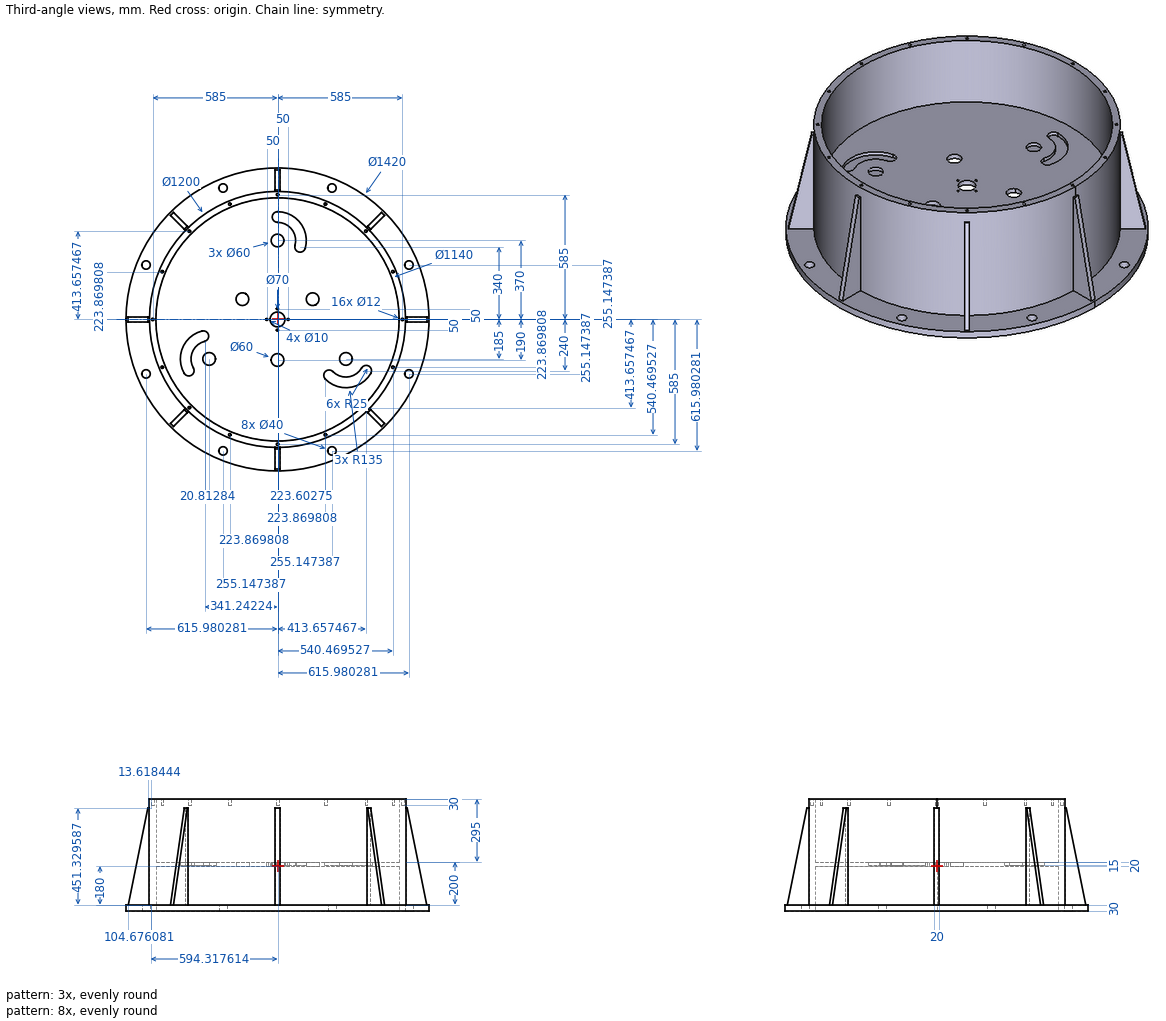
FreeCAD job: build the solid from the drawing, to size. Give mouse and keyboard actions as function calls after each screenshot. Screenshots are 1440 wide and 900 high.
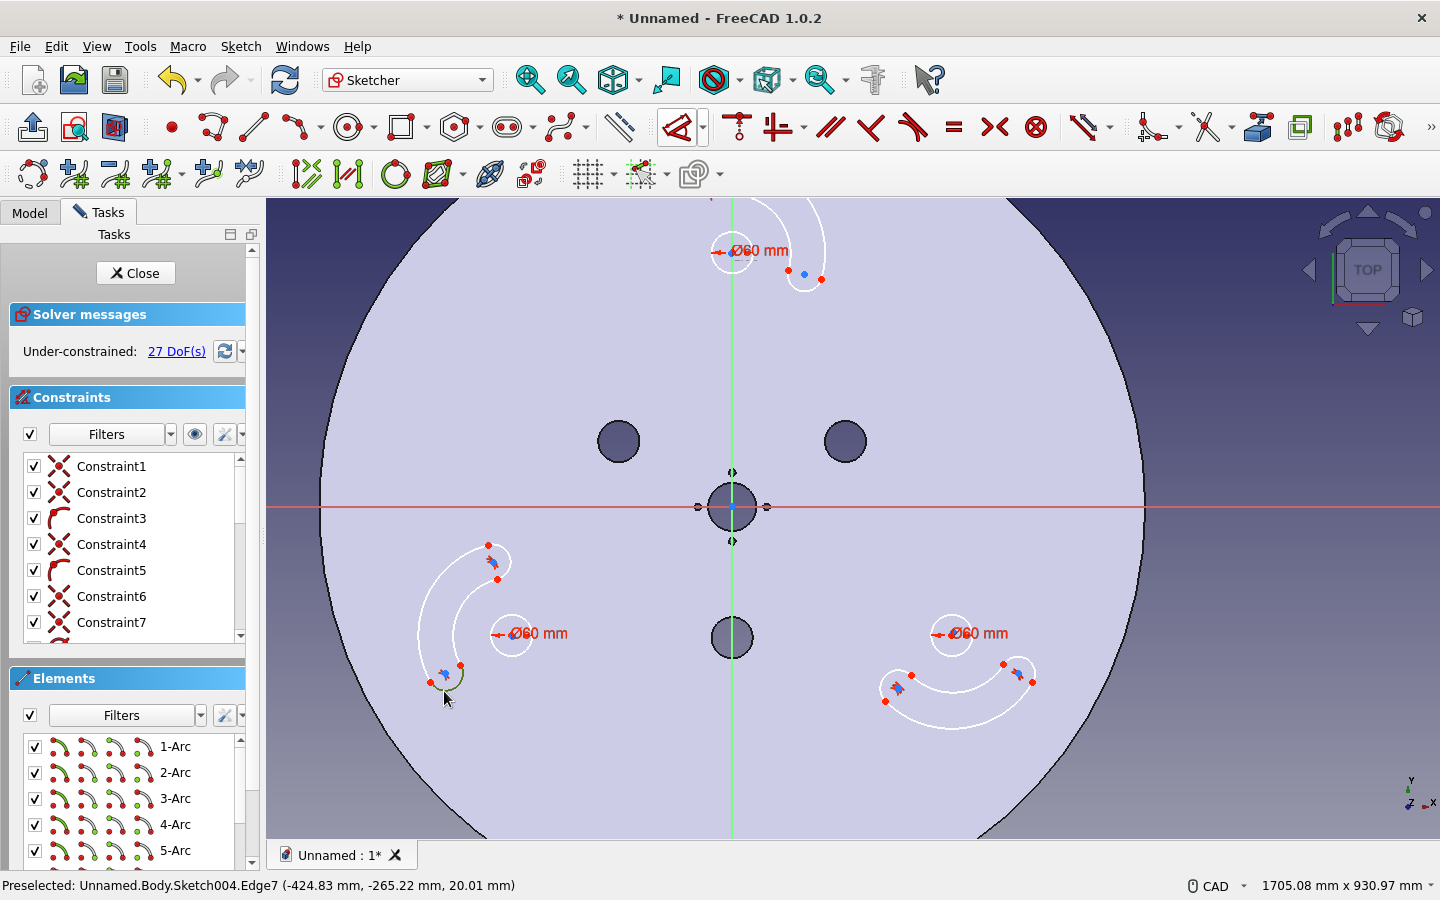
click(470, 595)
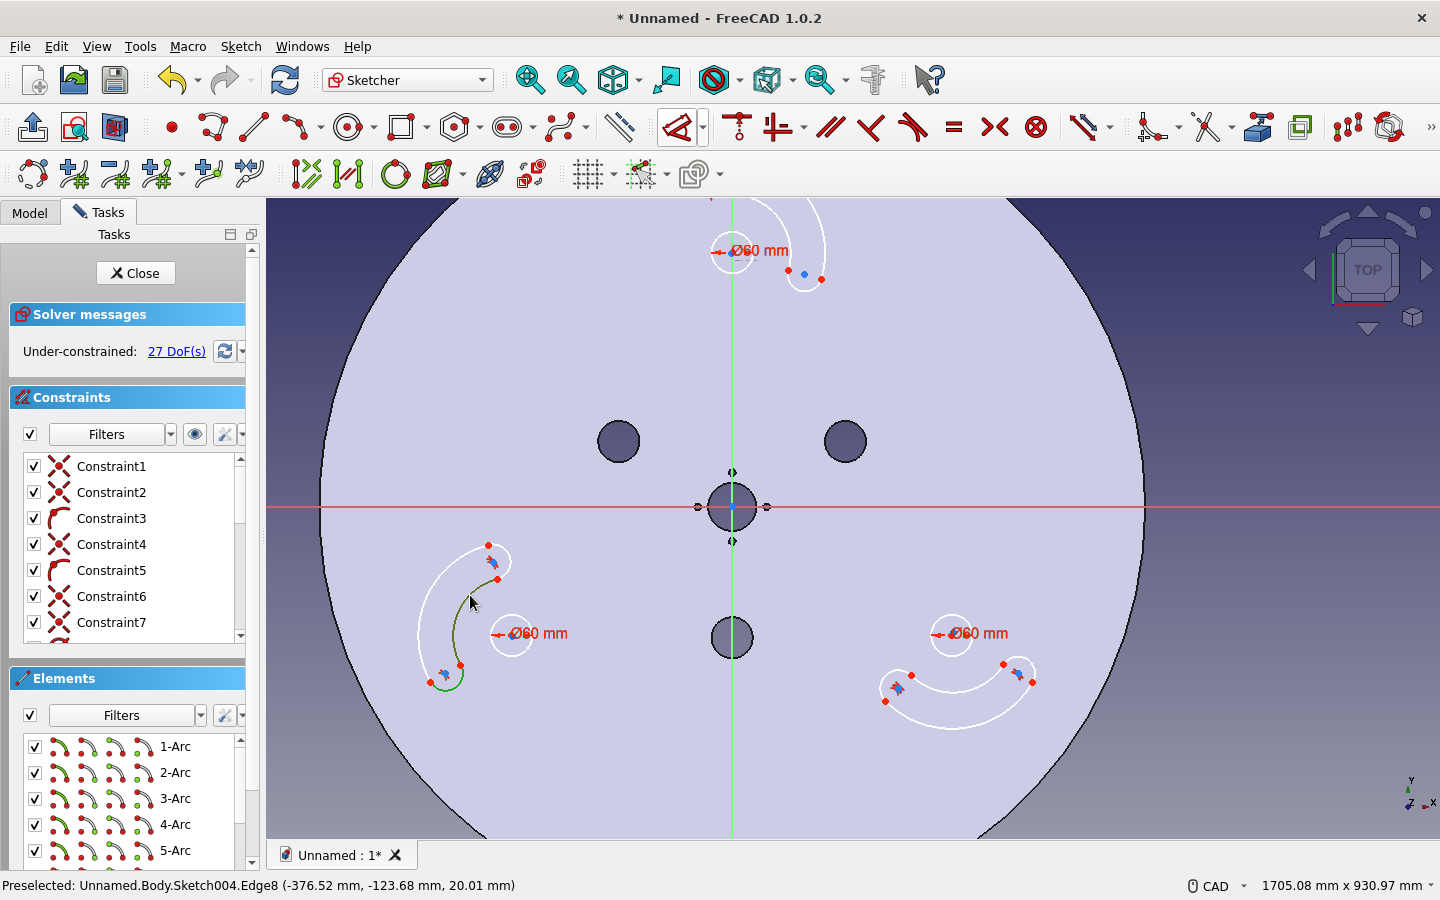
key(t)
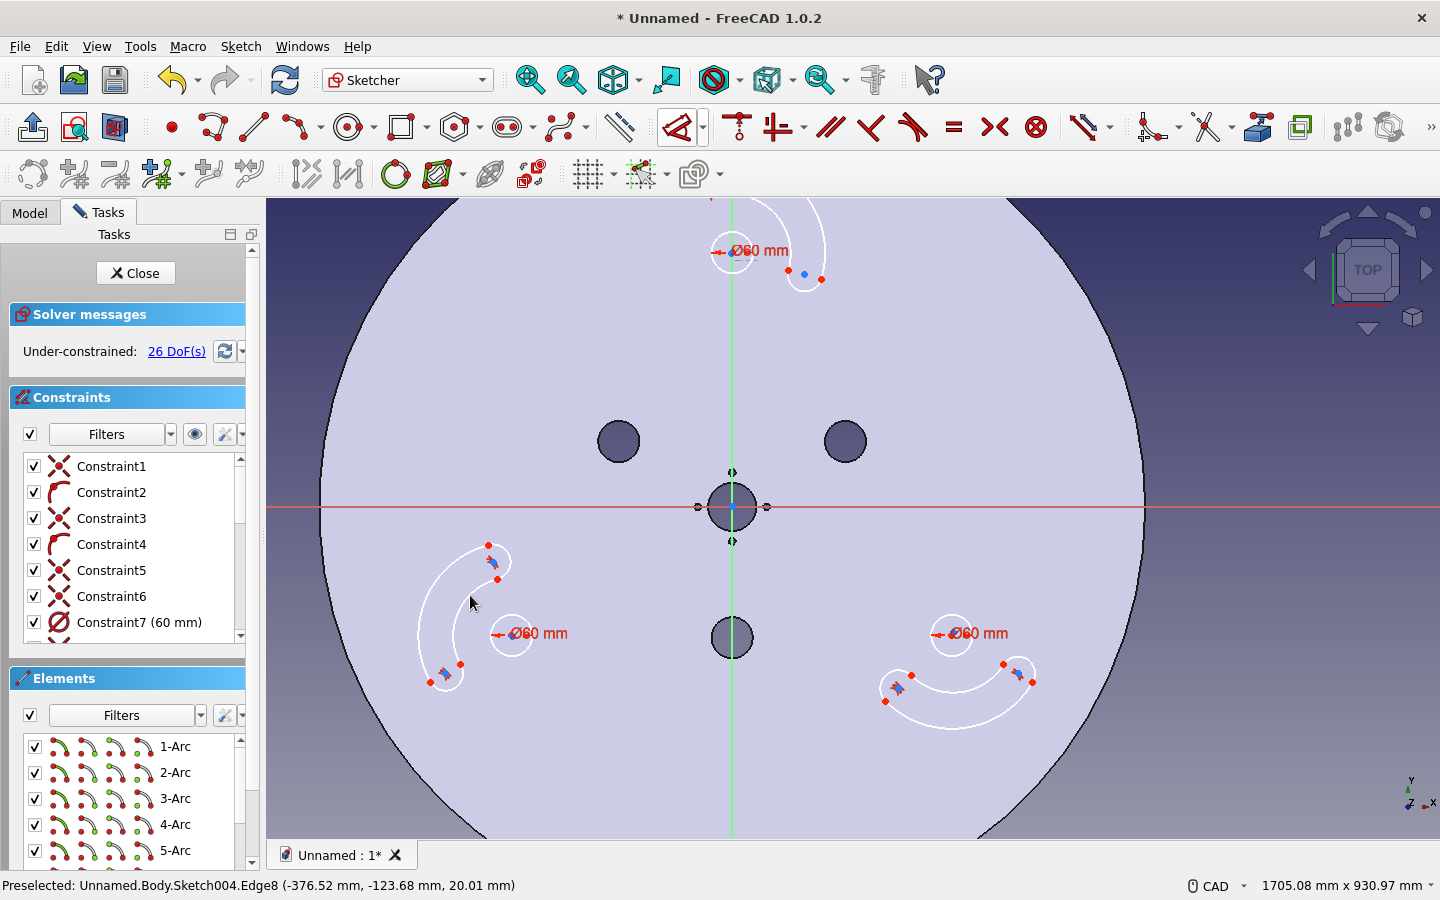
click(792, 285)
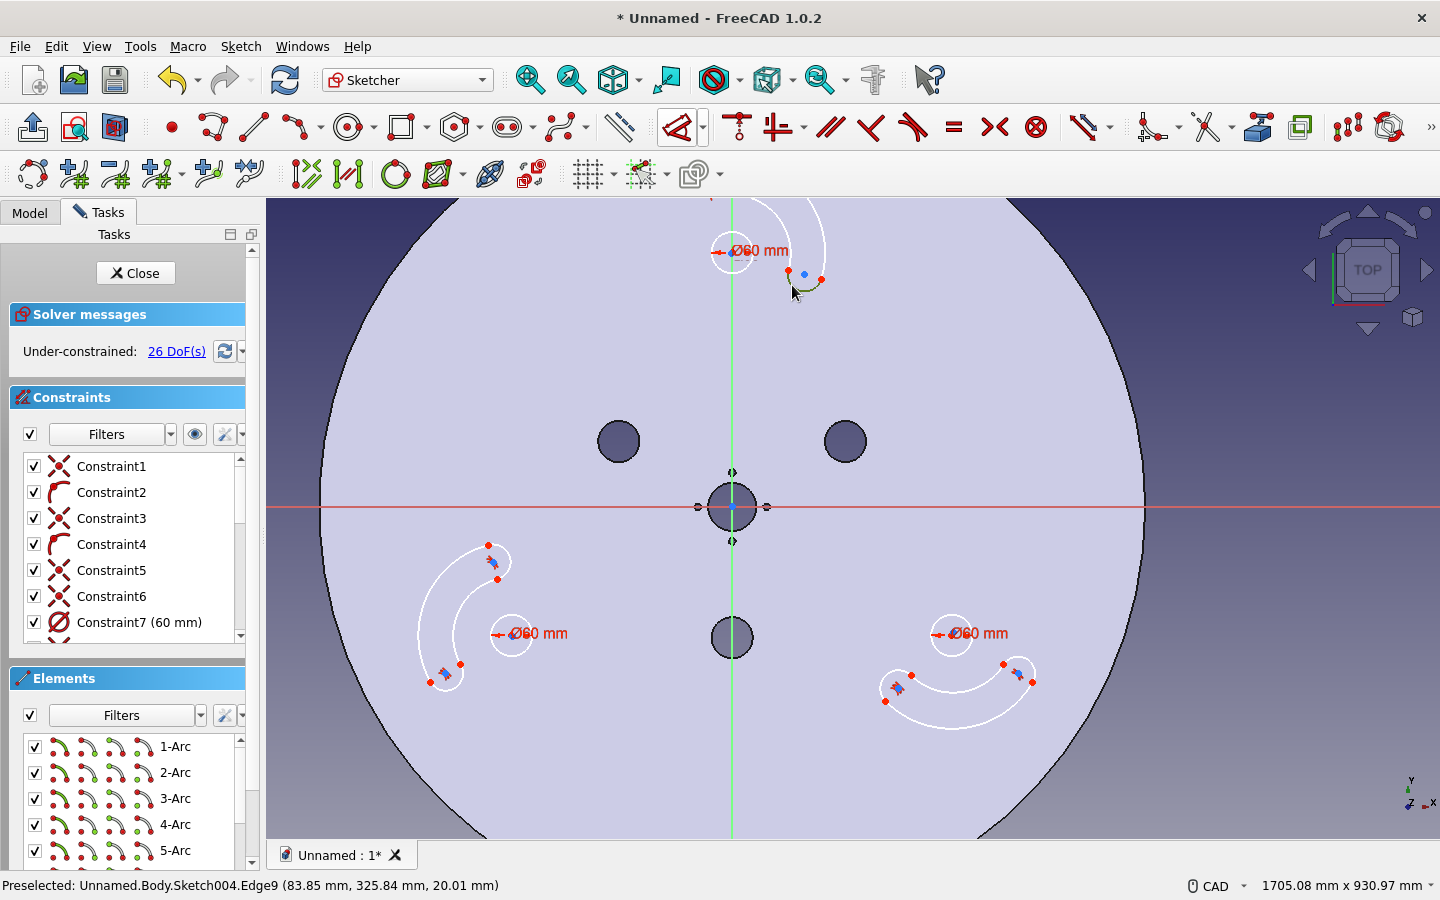
click(822, 228)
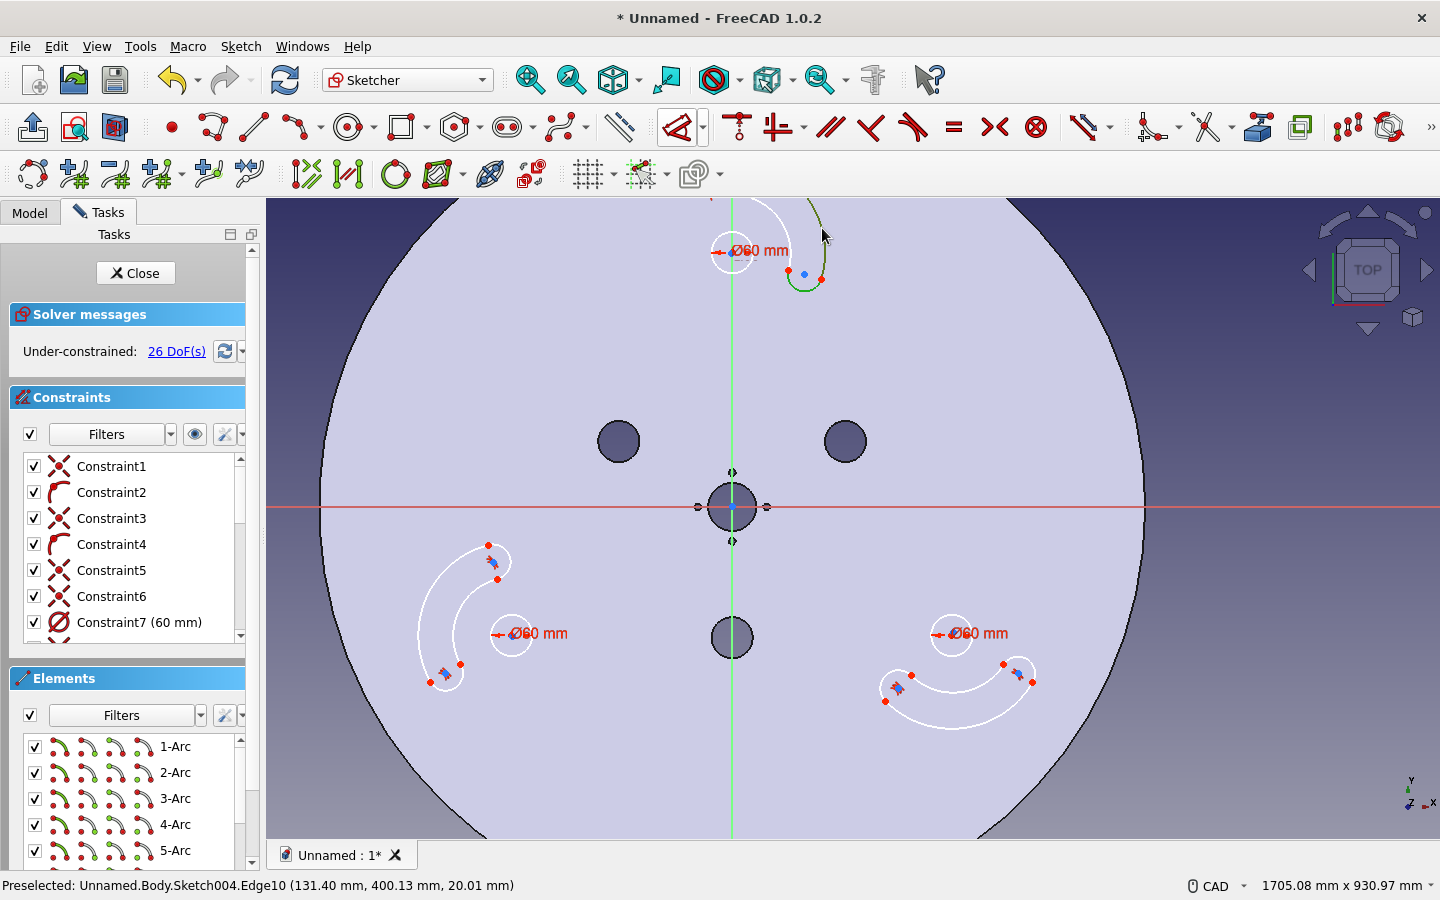
key(t)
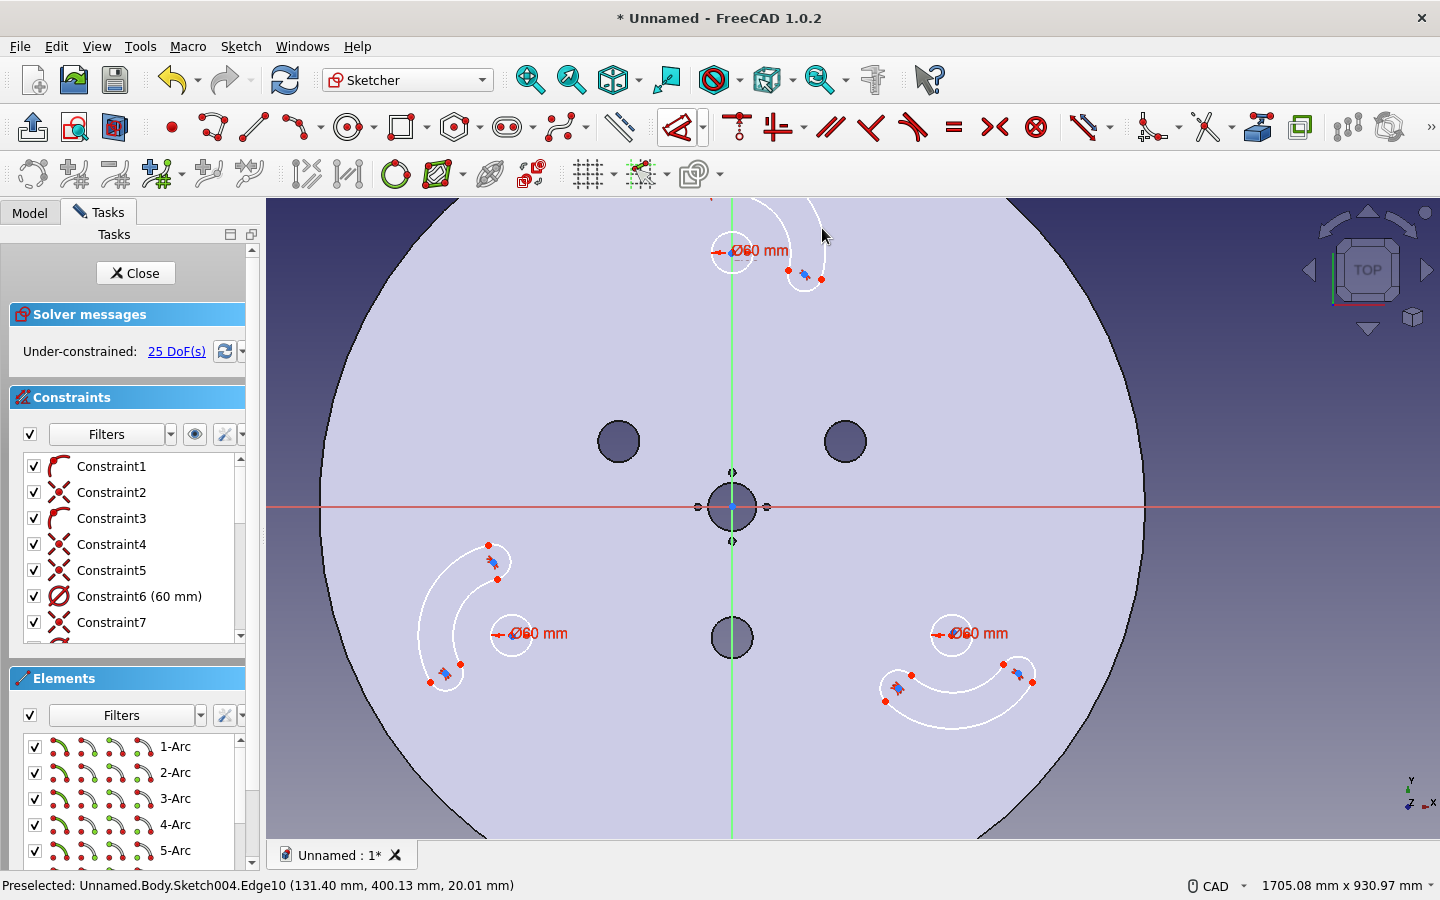
click(792, 285)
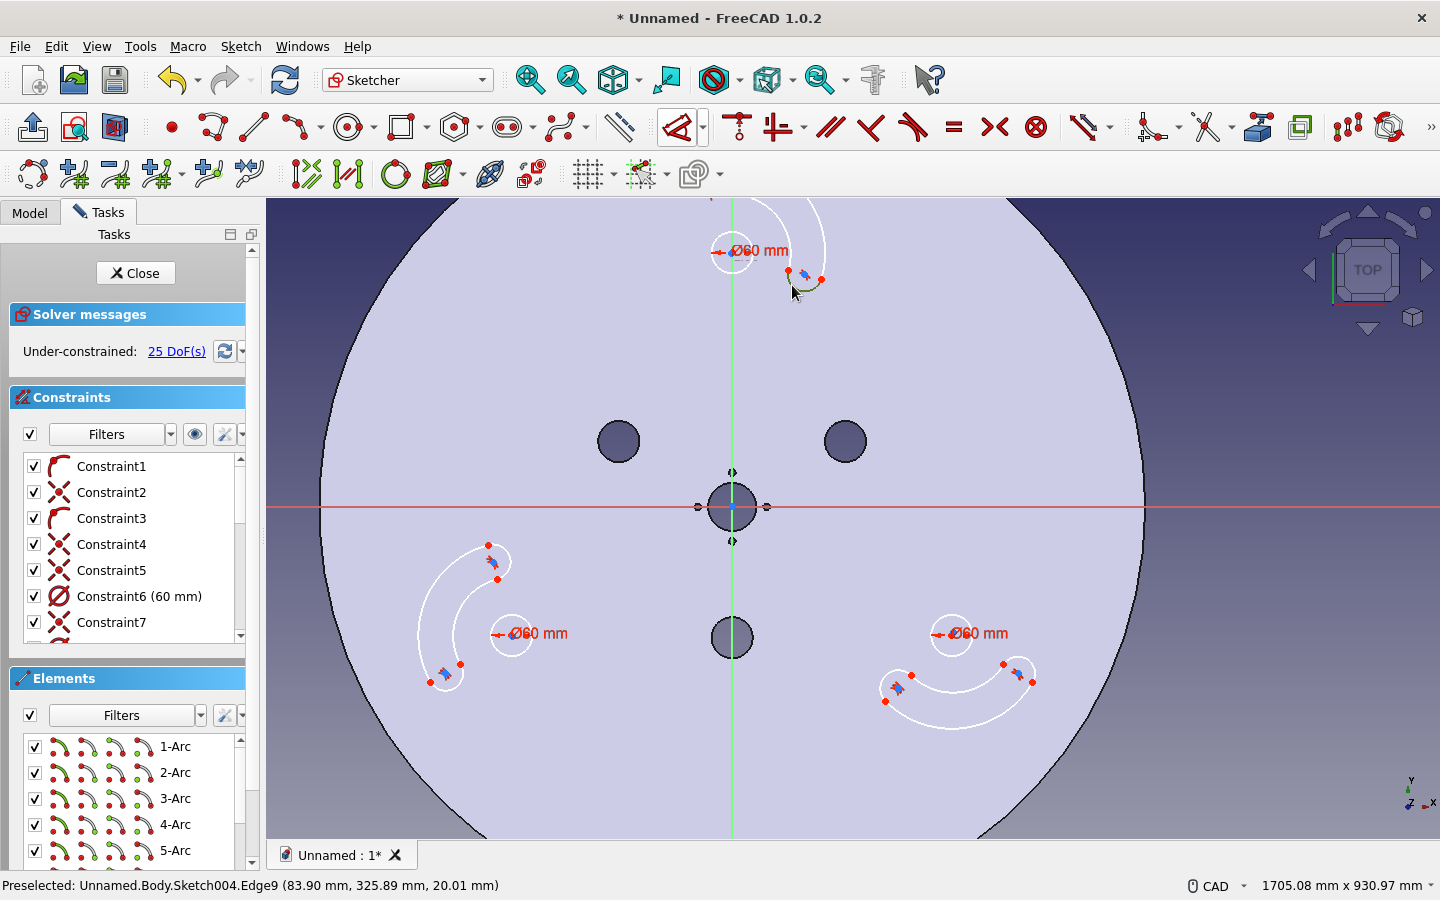
click(789, 238)